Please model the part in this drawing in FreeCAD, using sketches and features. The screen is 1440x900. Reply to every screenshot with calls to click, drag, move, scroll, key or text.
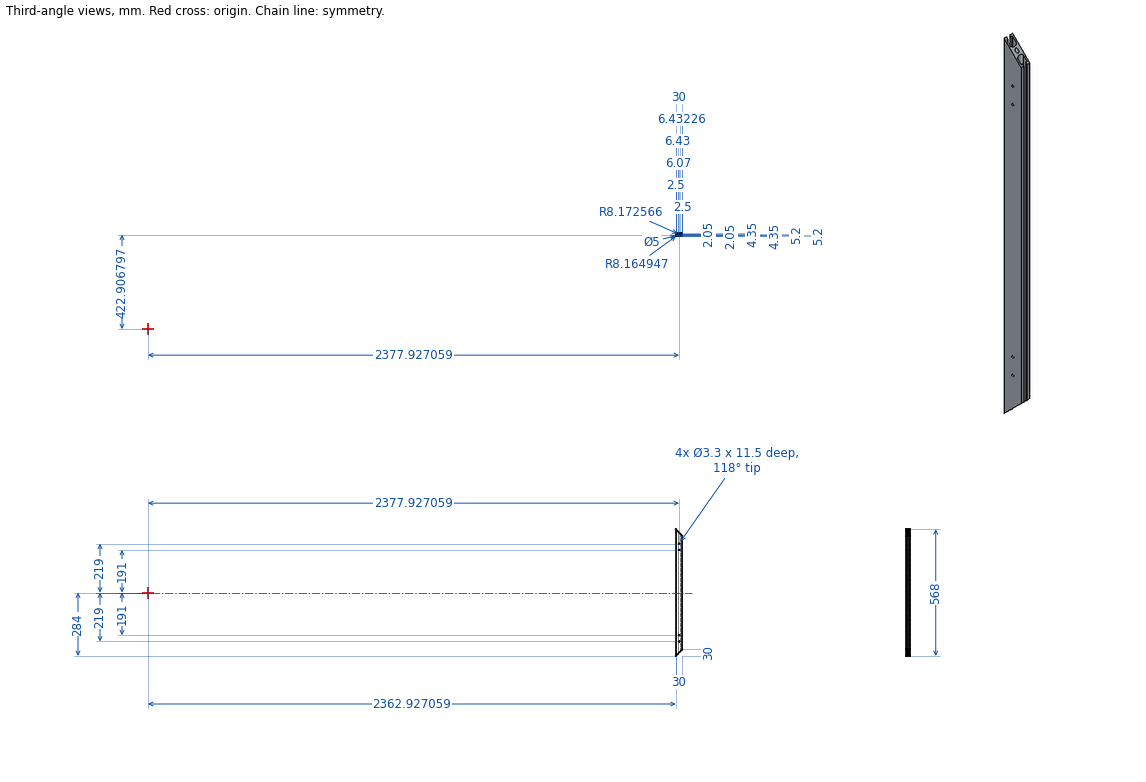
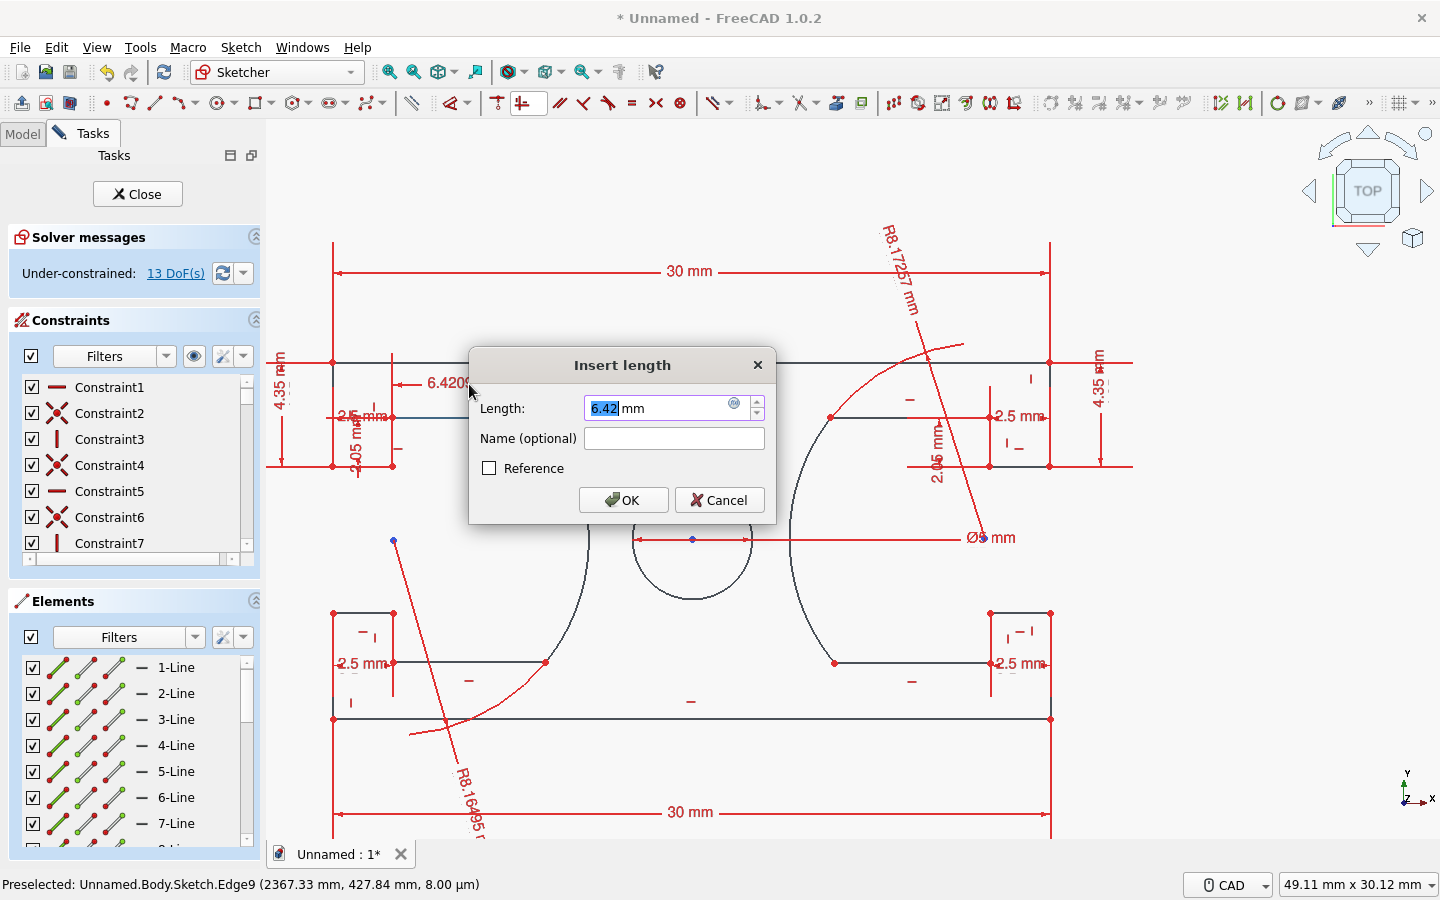
text(6.43)
key(Return)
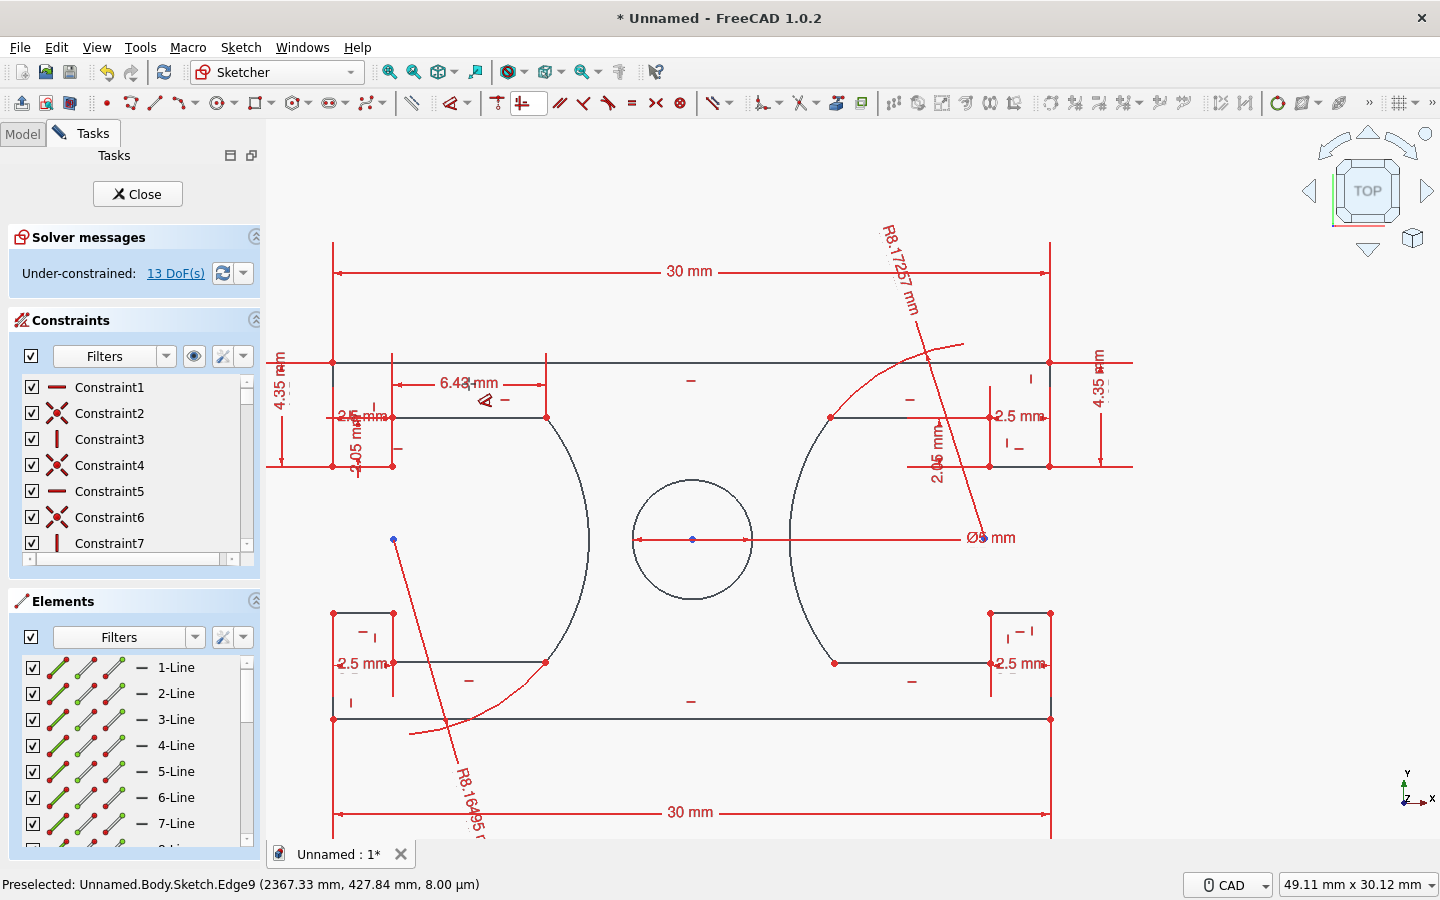
click(500, 662)
click(469, 696)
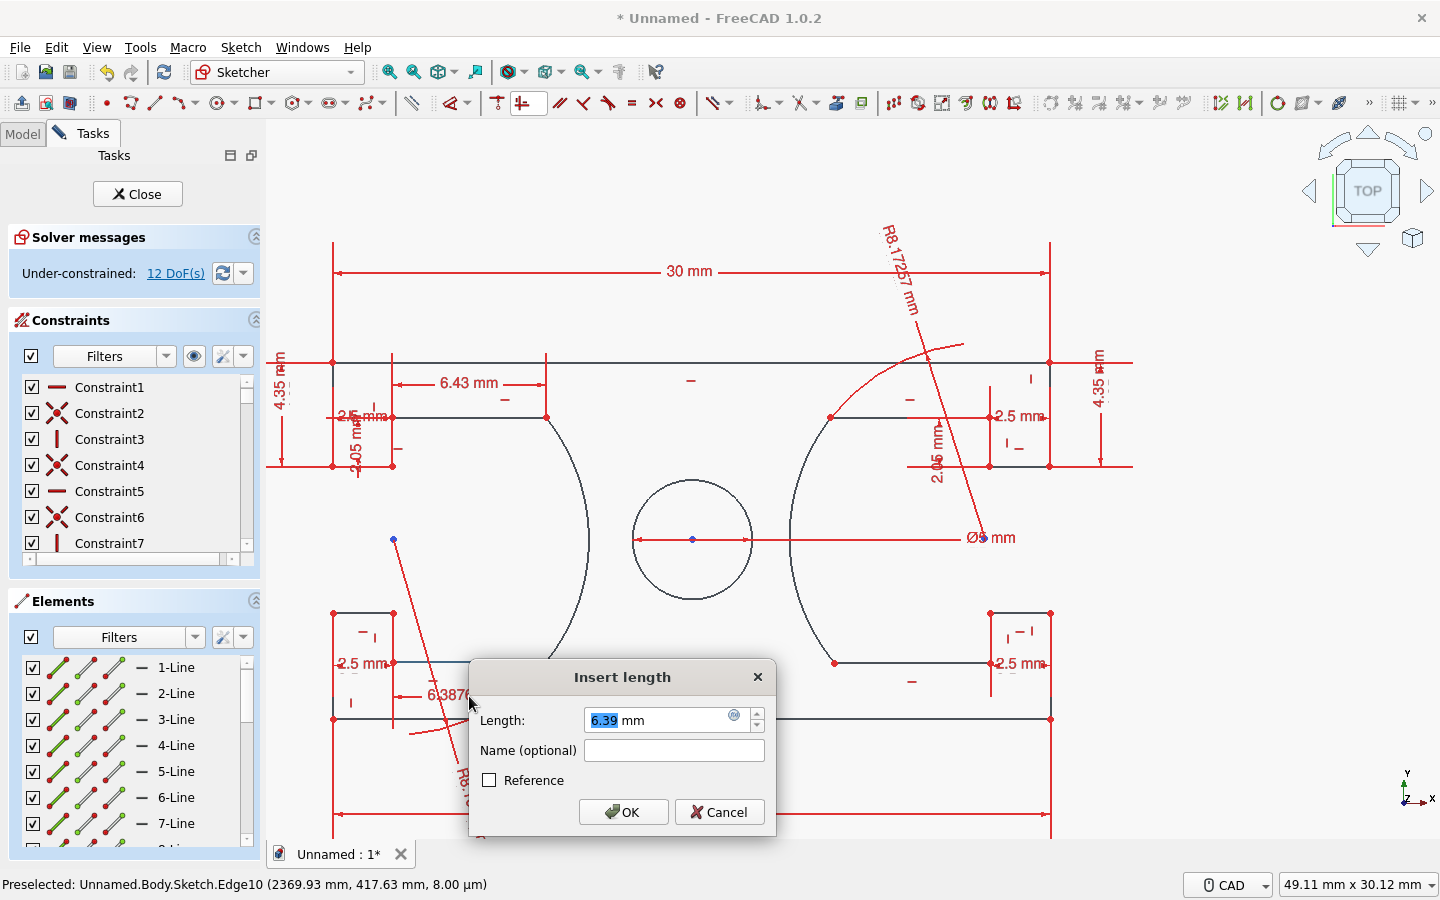
text(6.43)
key(Return)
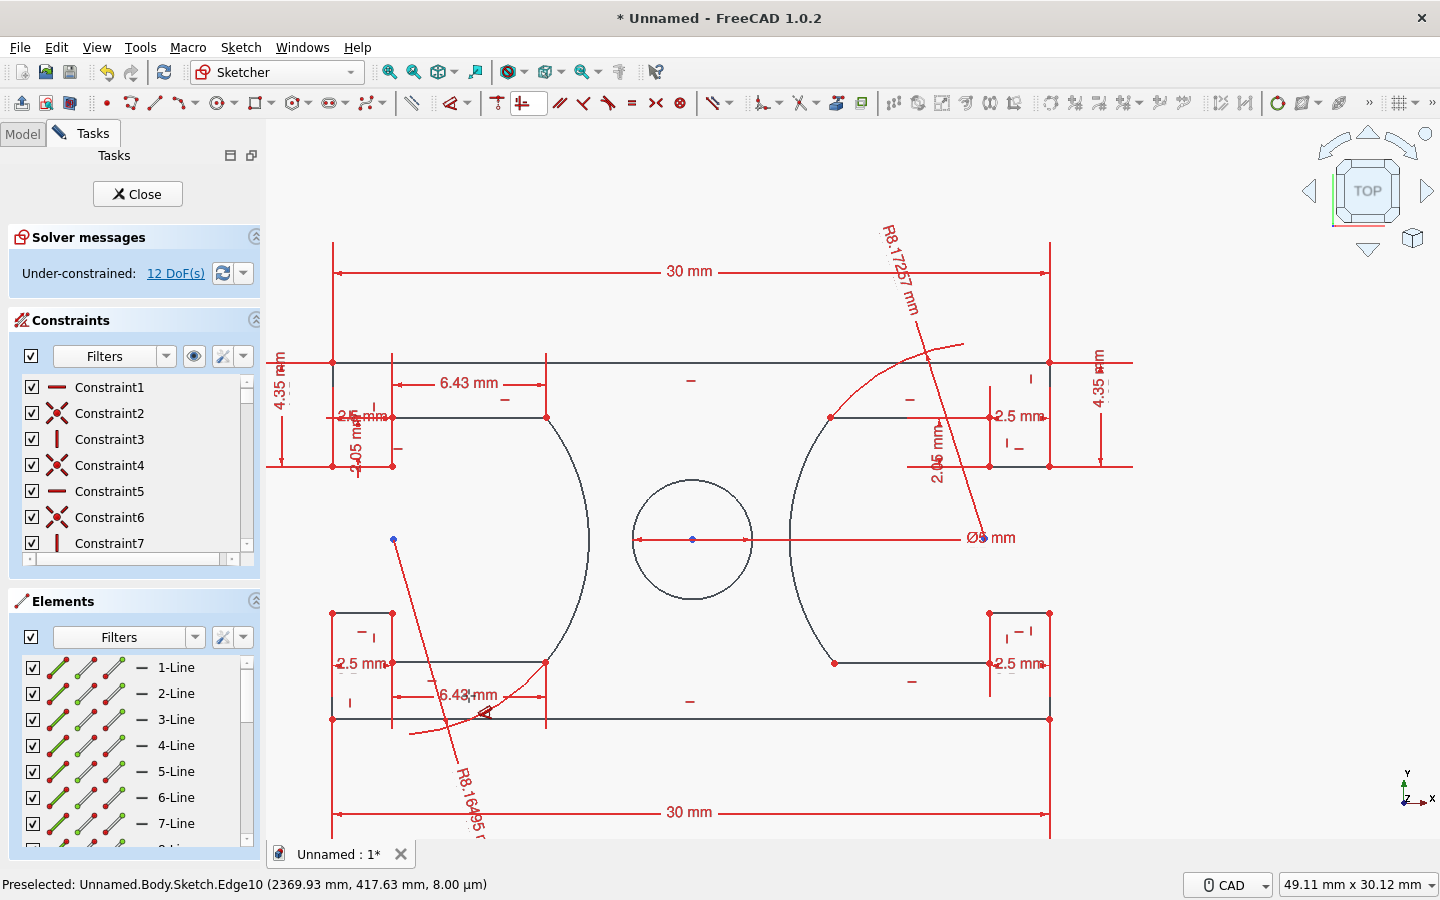
click(392, 647)
click(358, 638)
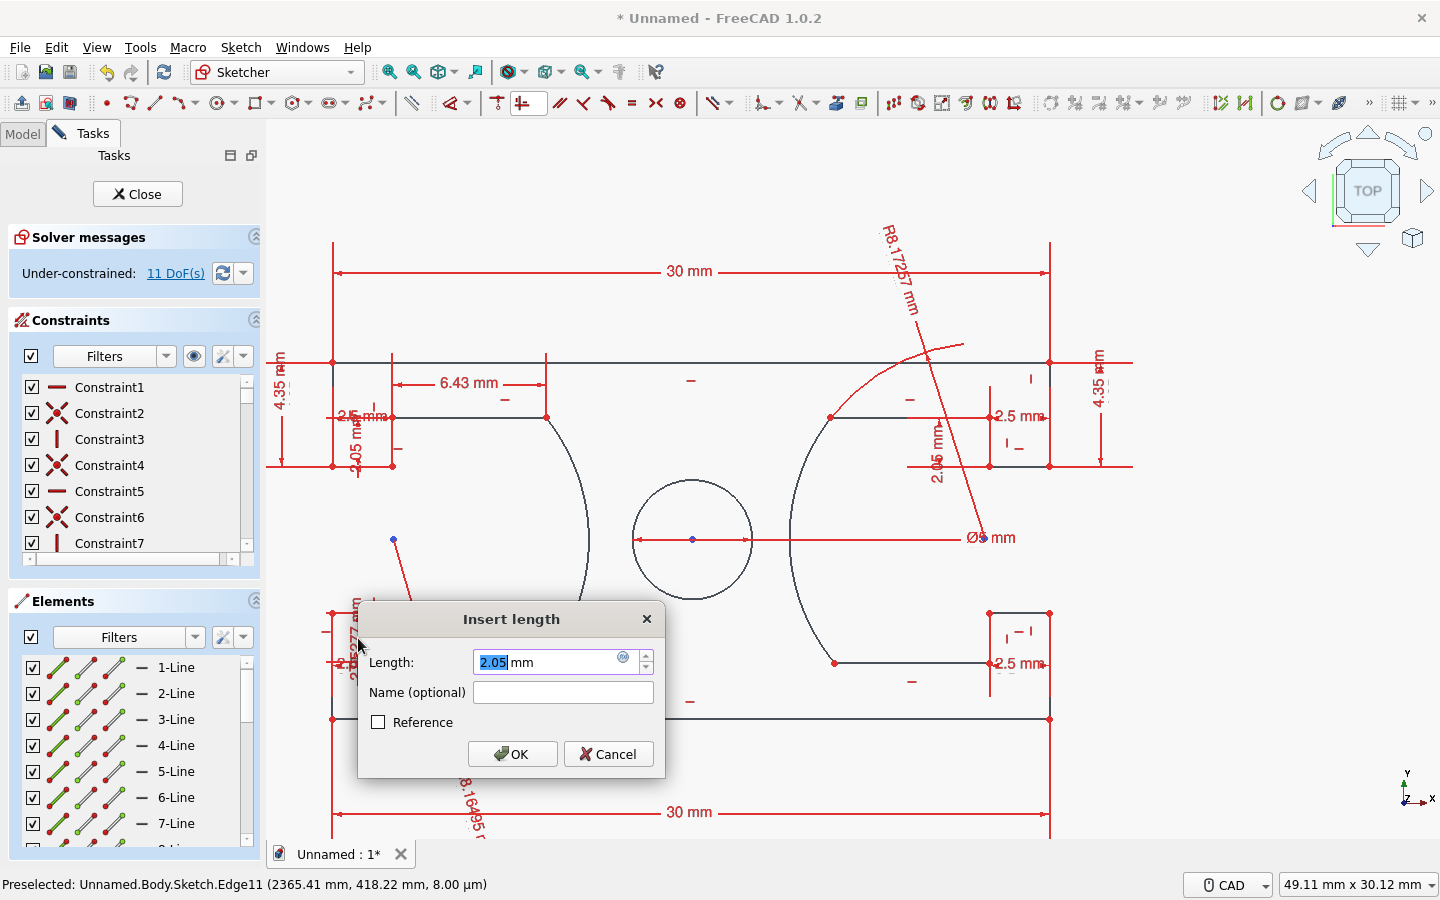
text(2.05)
key(Return)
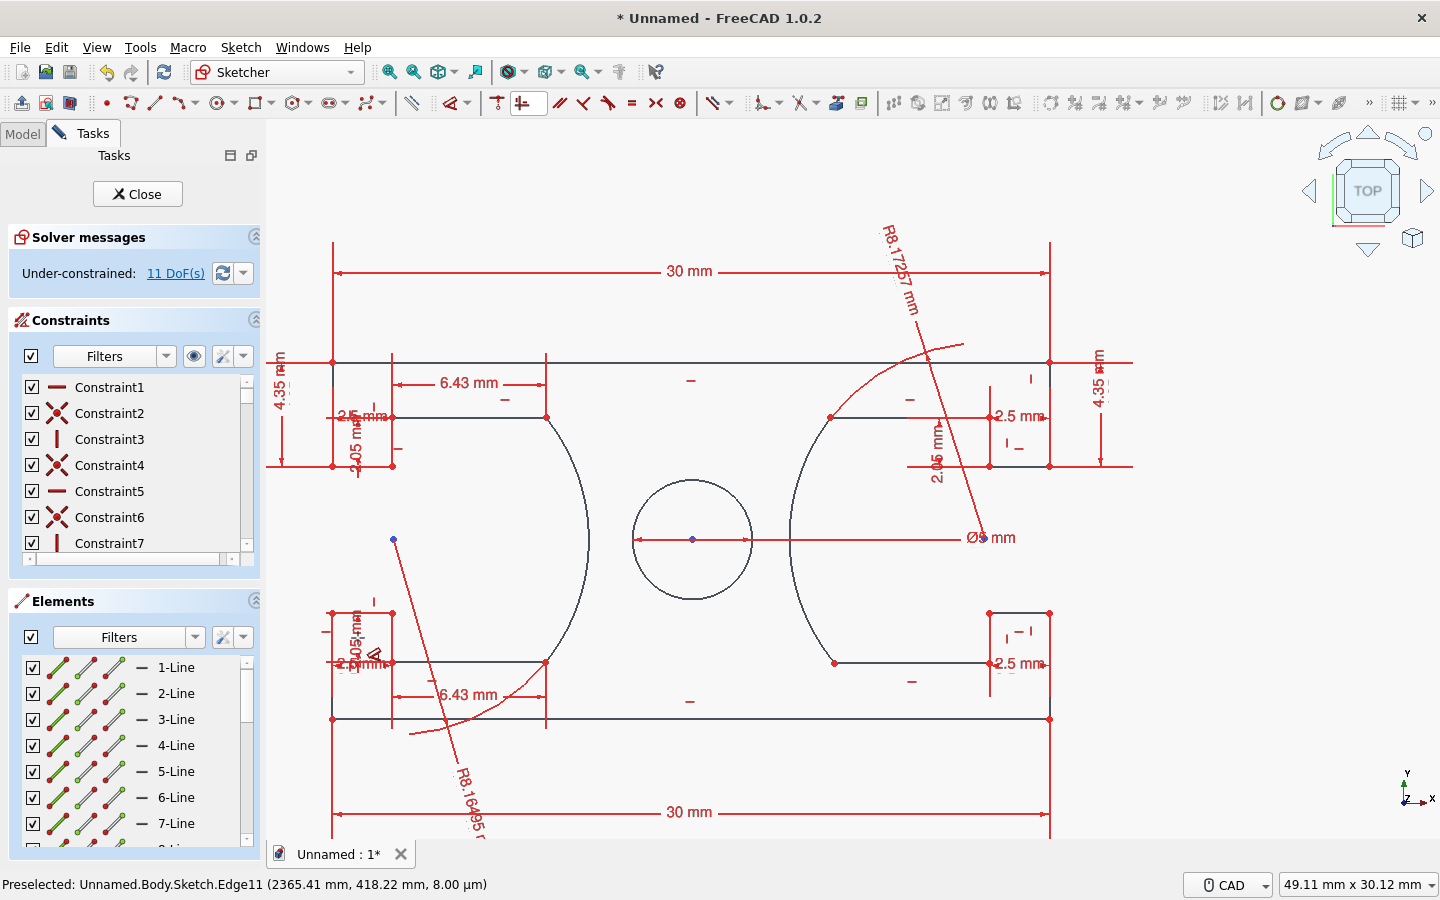
click(332, 645)
click(298, 691)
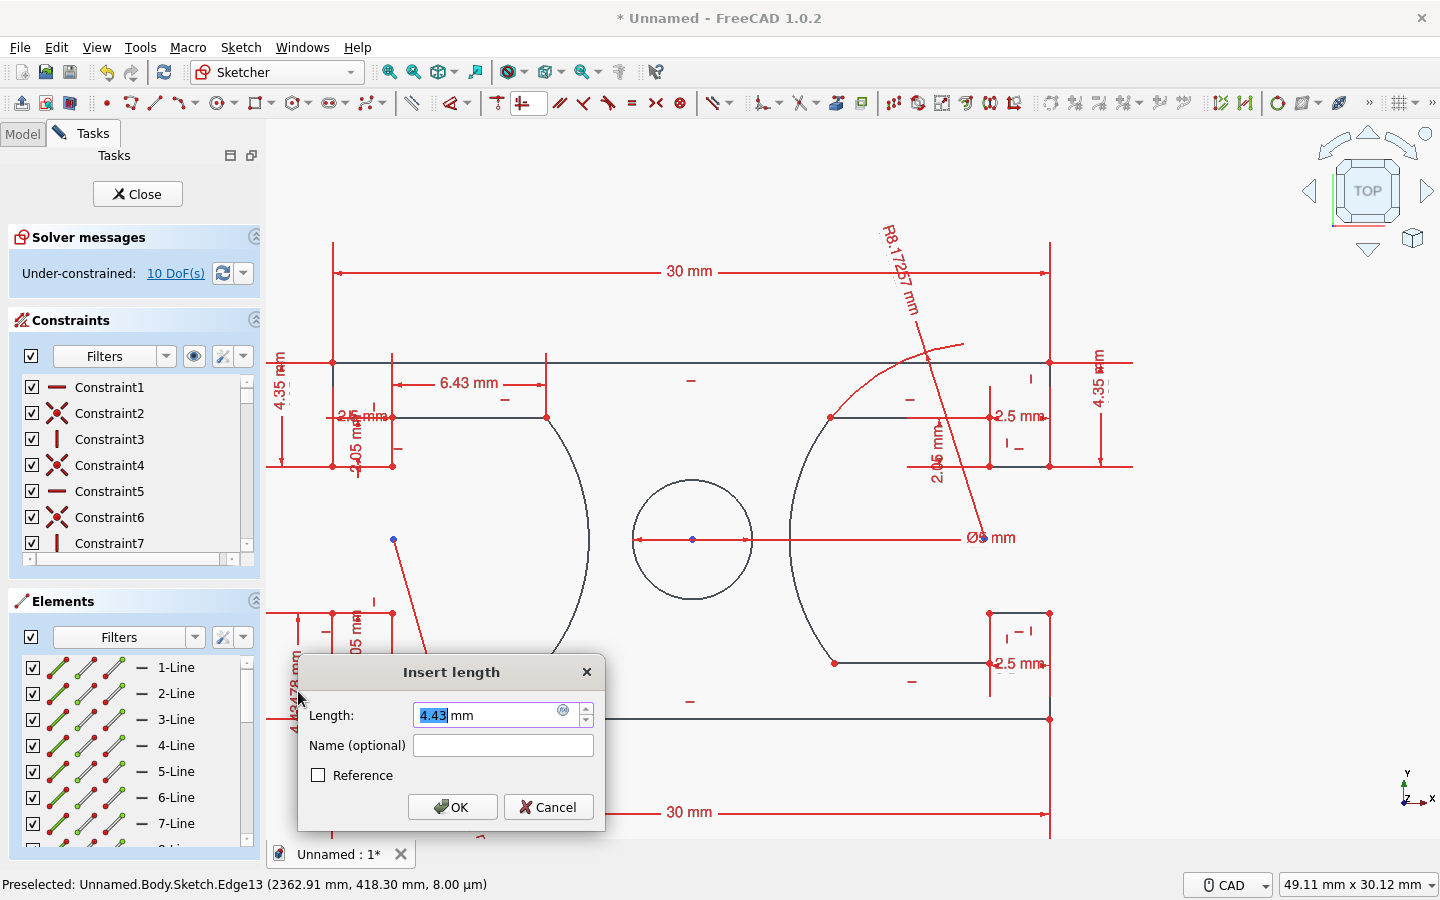
text(4.35)
key(Return)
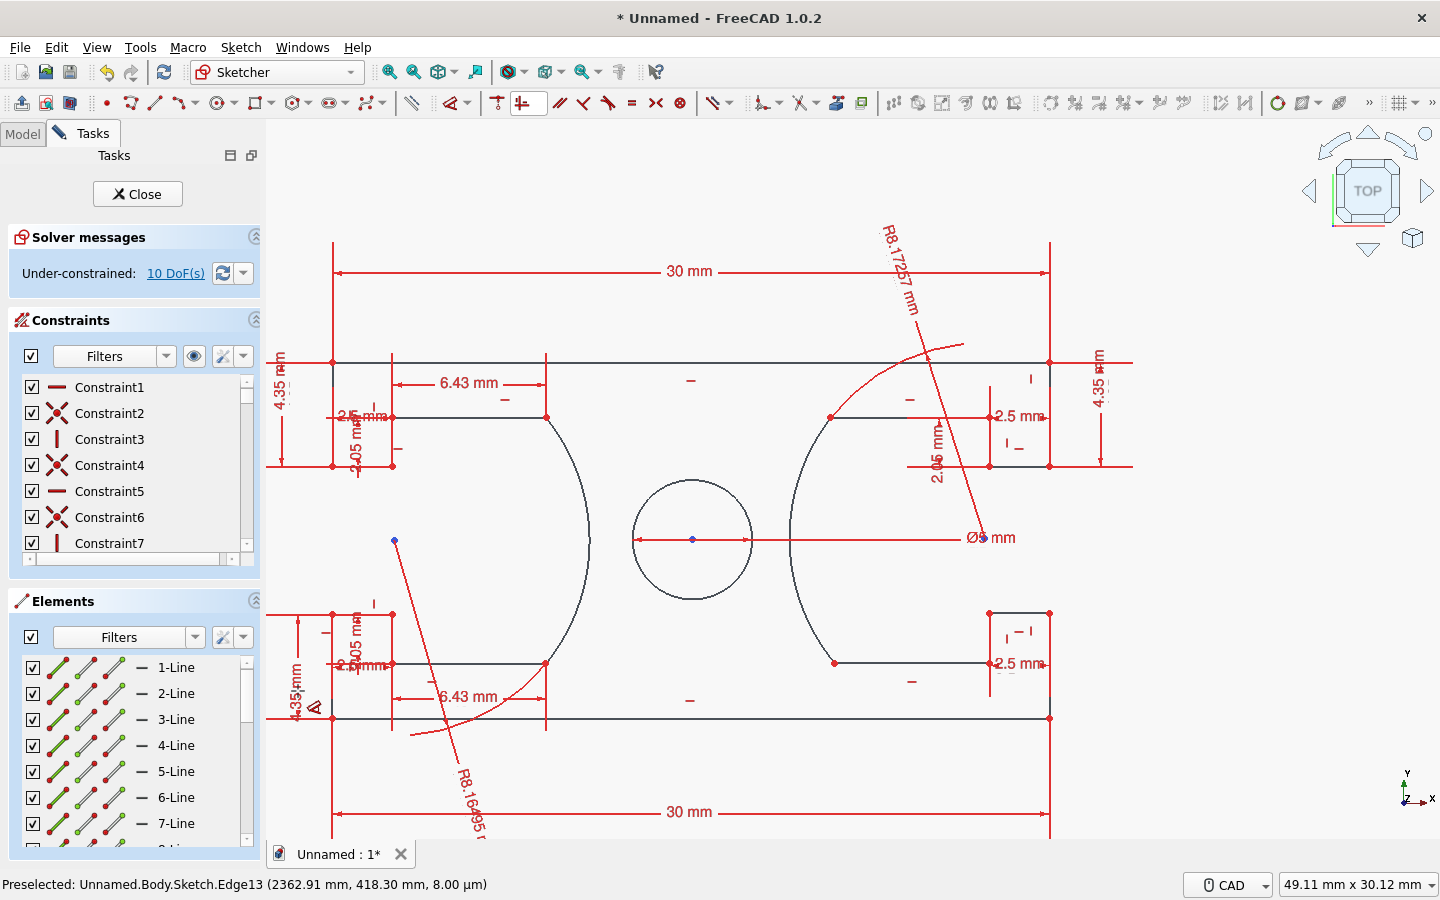
click(1050, 687)
click(1084, 642)